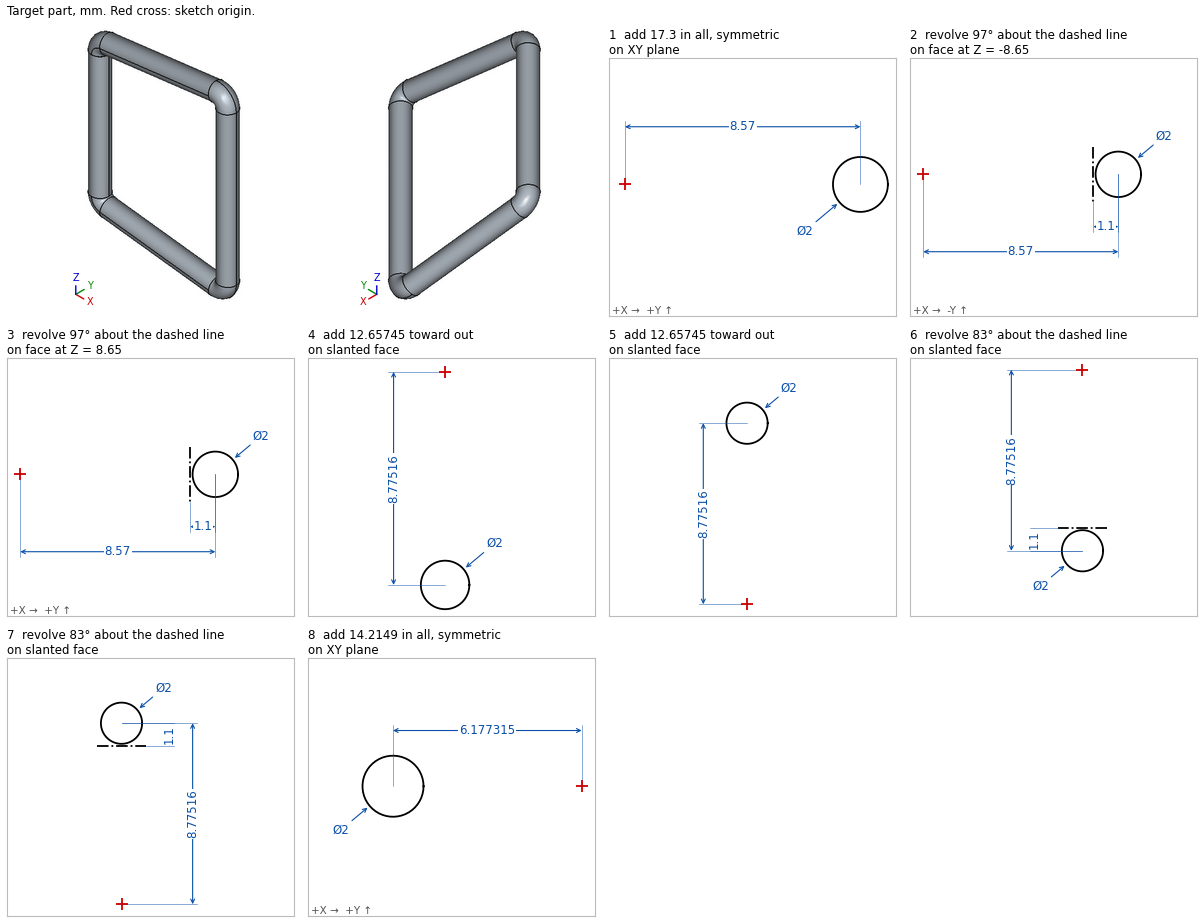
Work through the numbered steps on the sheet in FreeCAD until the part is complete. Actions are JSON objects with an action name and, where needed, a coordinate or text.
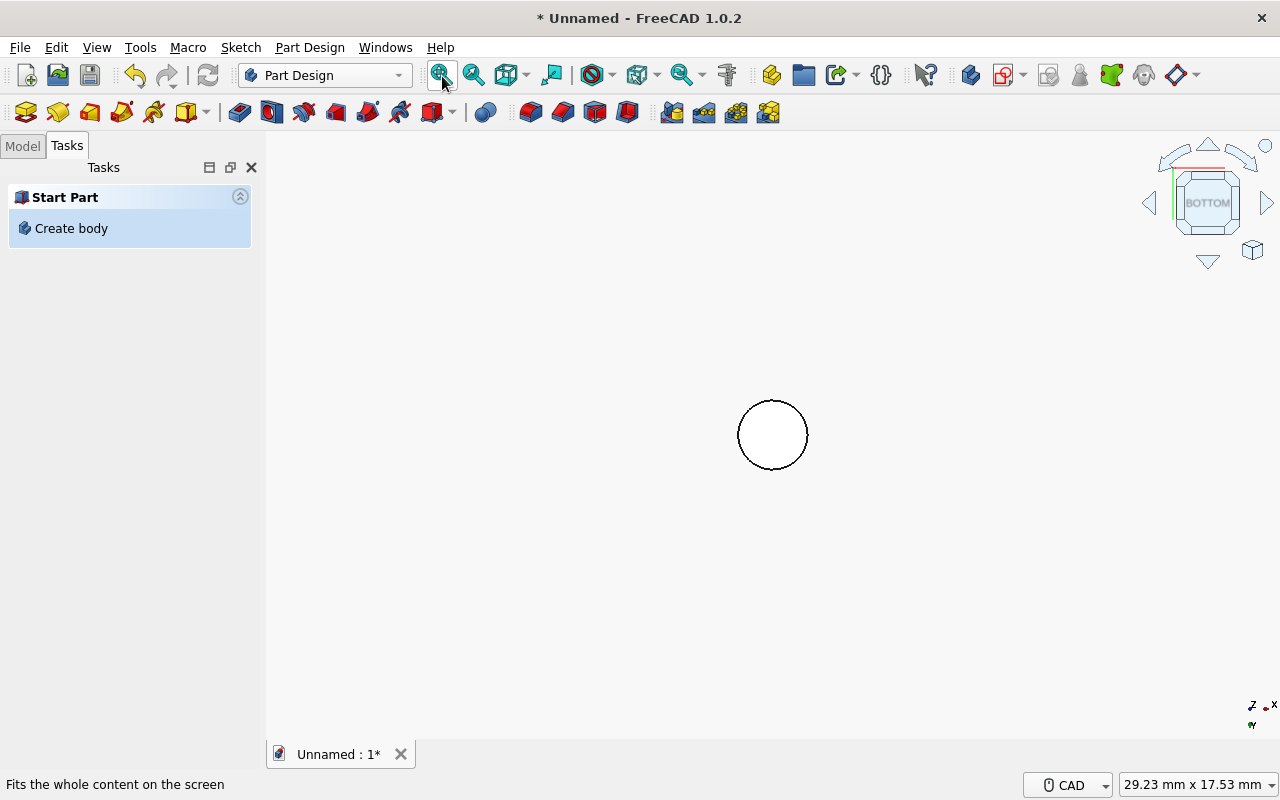
{"action": "left_click", "coordinate": [773, 434]}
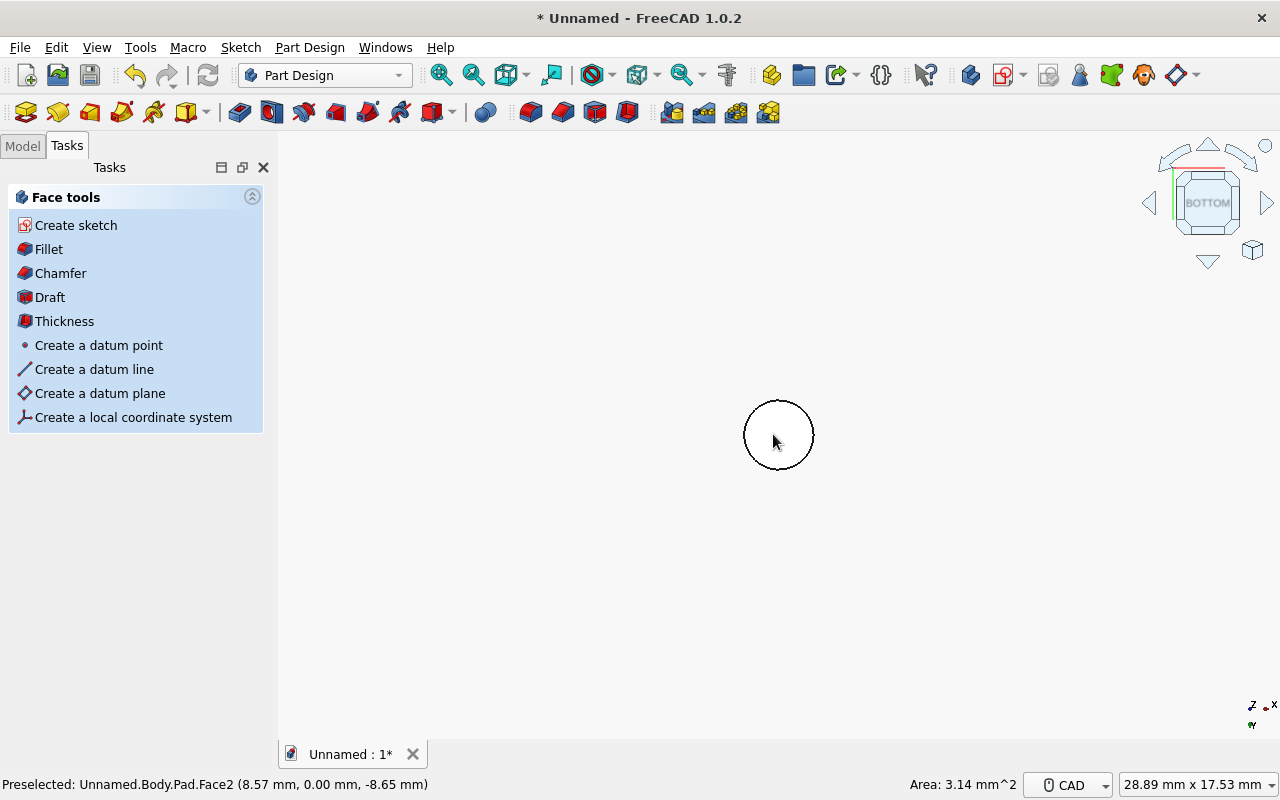
{"action": "left_click", "coordinate": [1004, 76]}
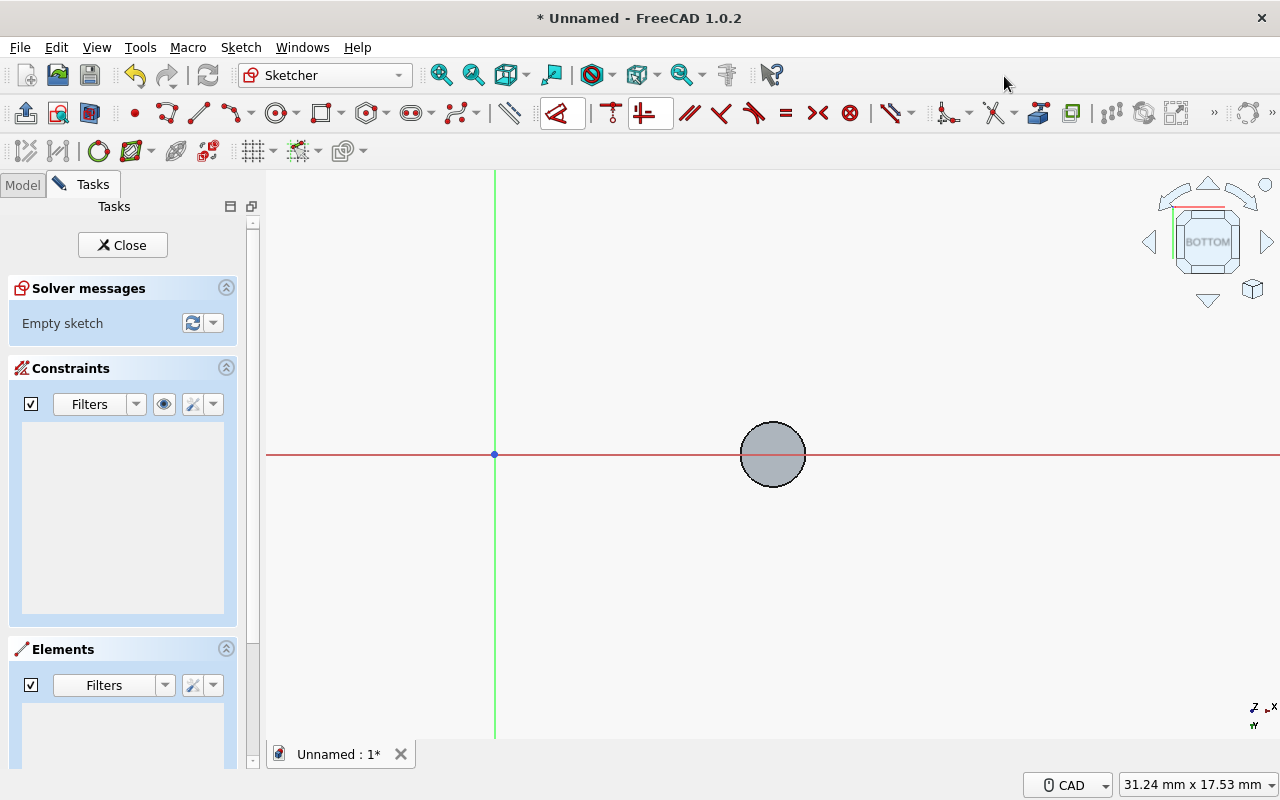
{"action": "scroll", "coordinate": [788, 454], "scroll_direction": "up", "scroll_amount": 8}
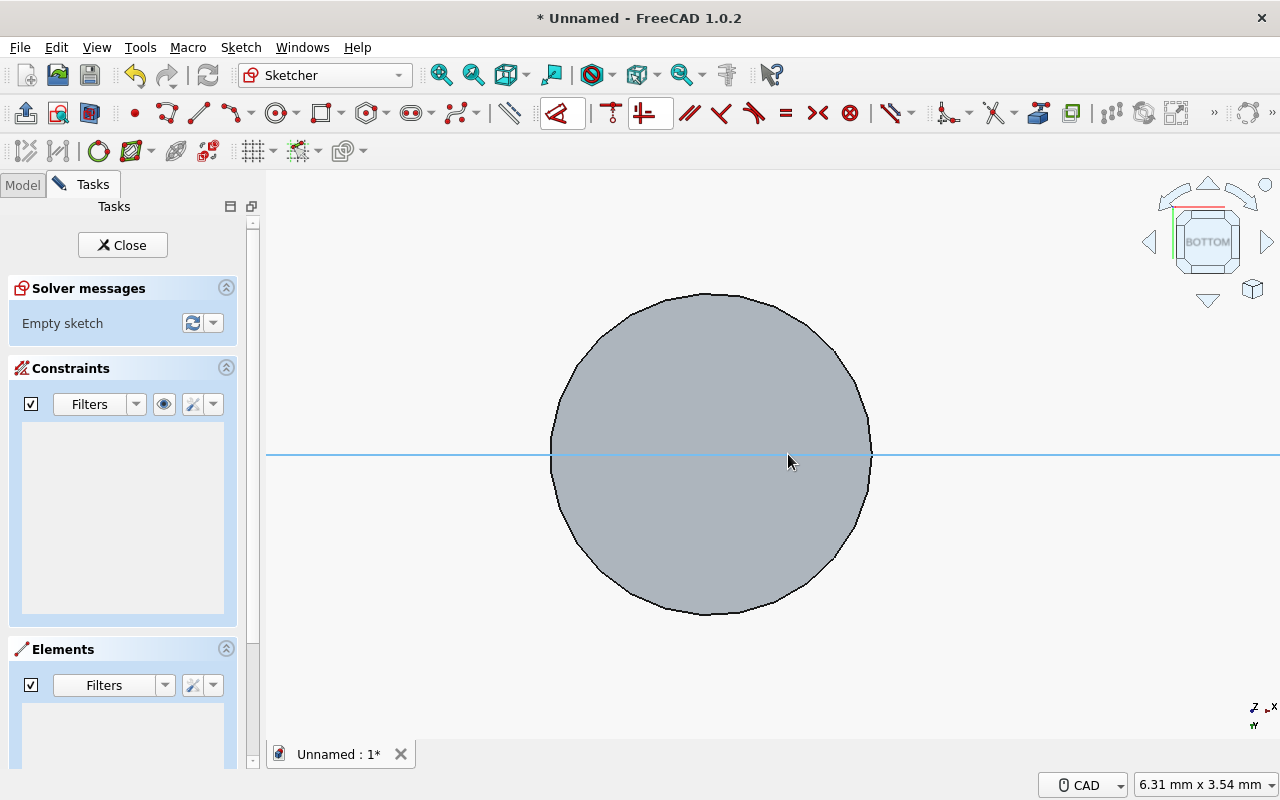
{"action": "key", "text": "g c"}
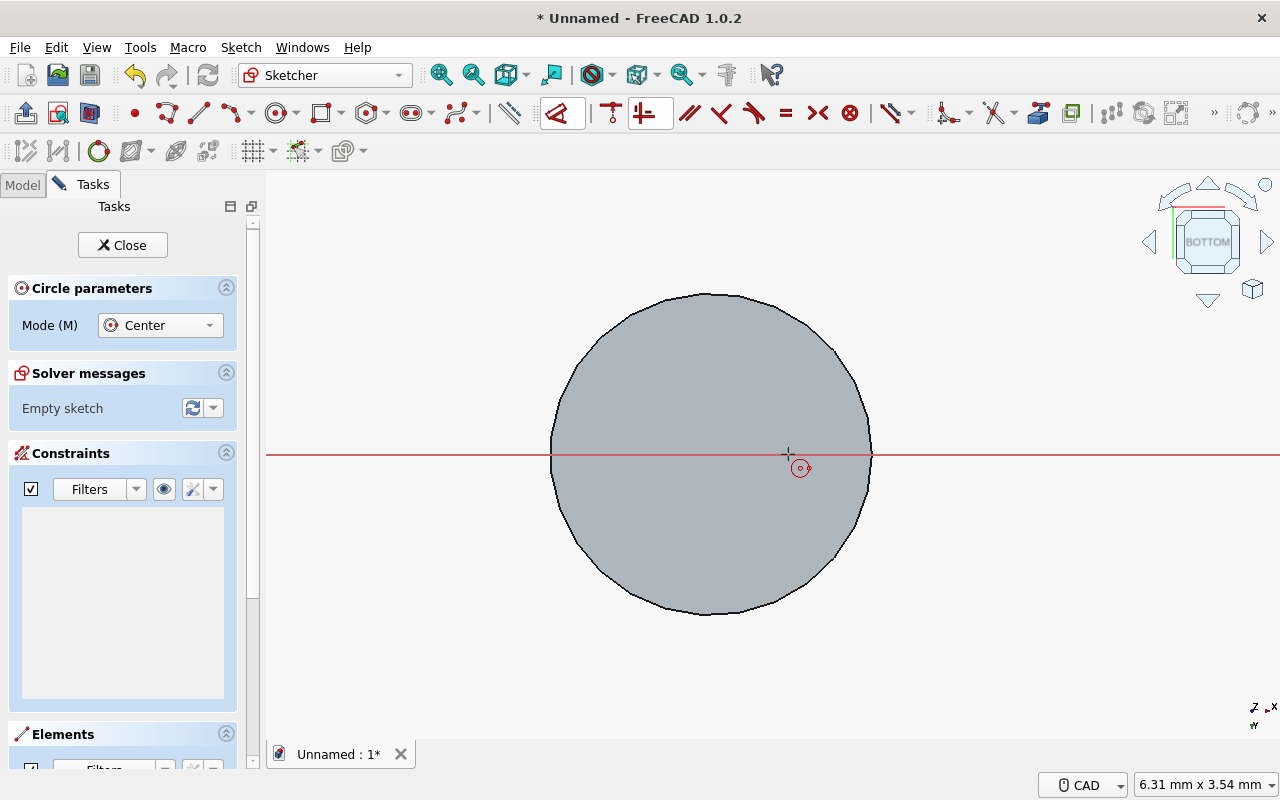
{"action": "left_click", "coordinate": [711, 454]}
{"action": "mouse_move", "coordinate": [825, 341]}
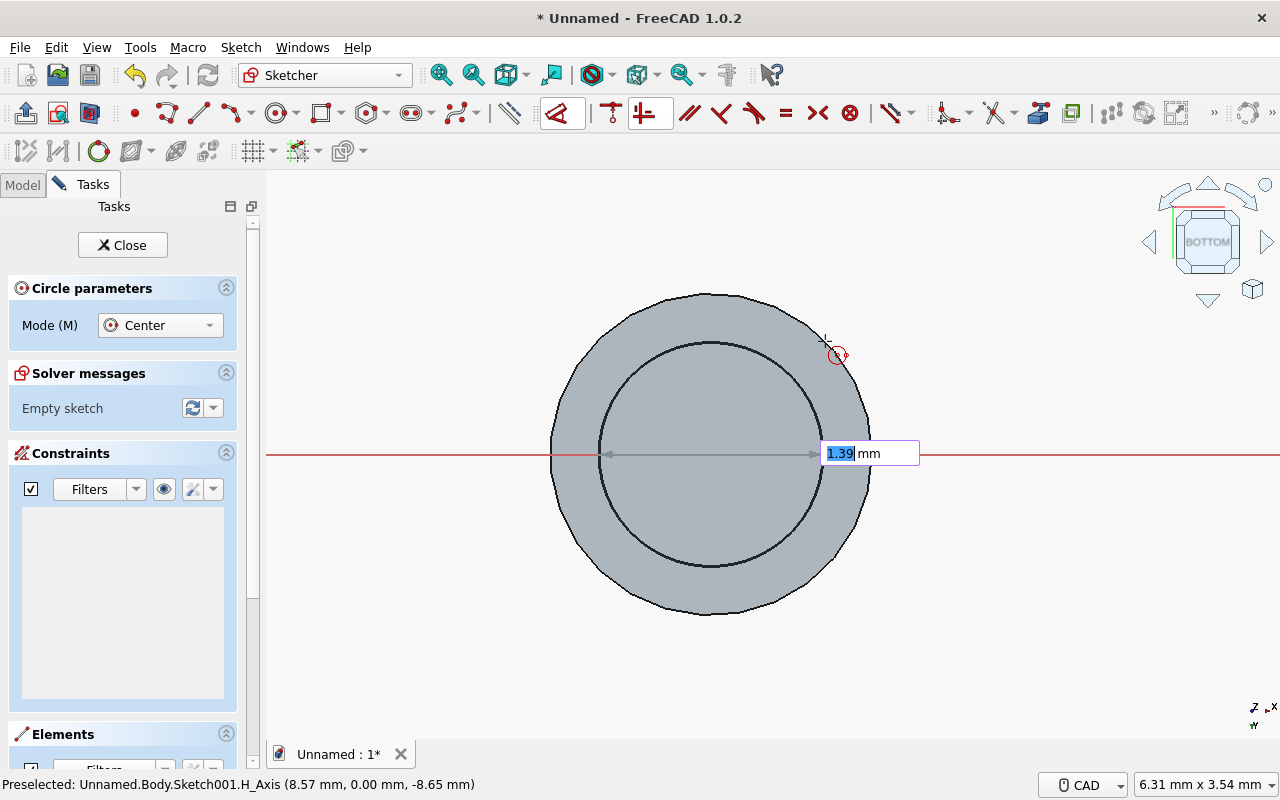
{"action": "type", "text": "2"}
{"action": "key", "text": "Return"}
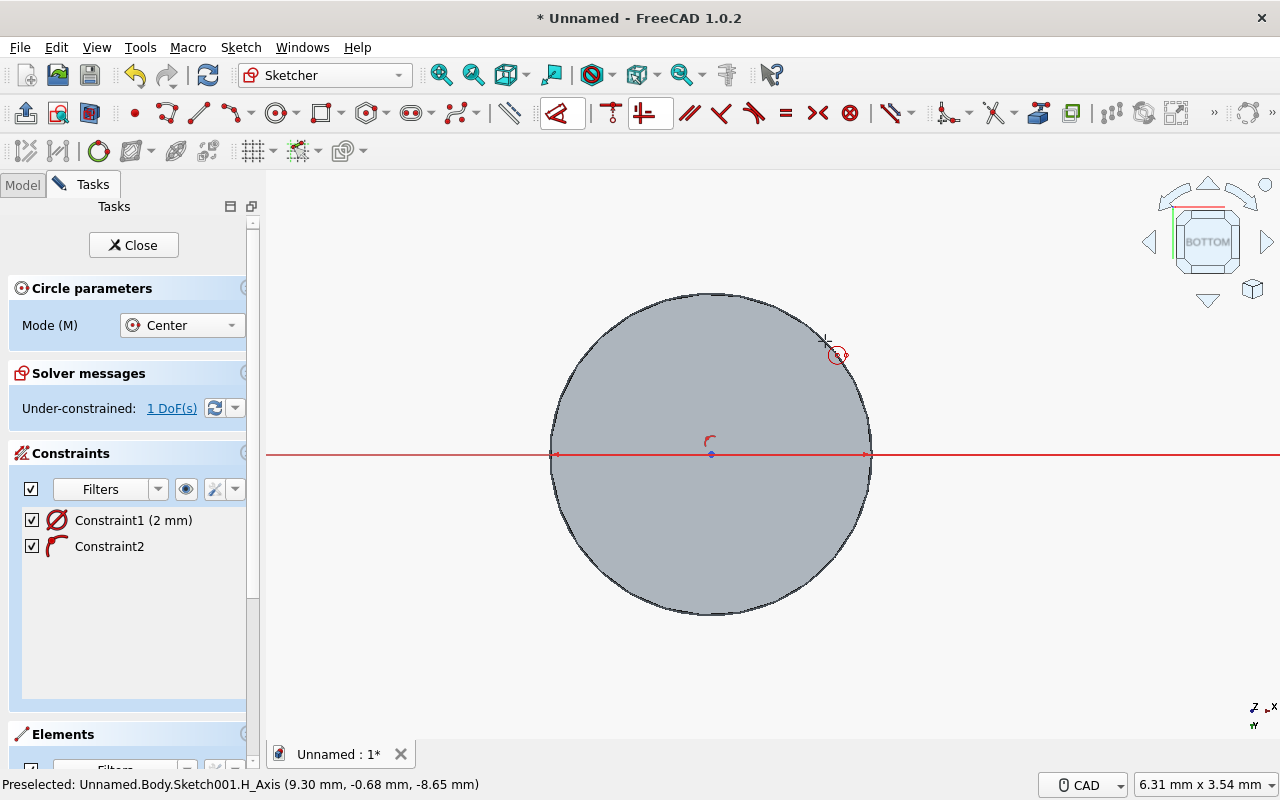
{"action": "left_click", "coordinate": [200, 114]}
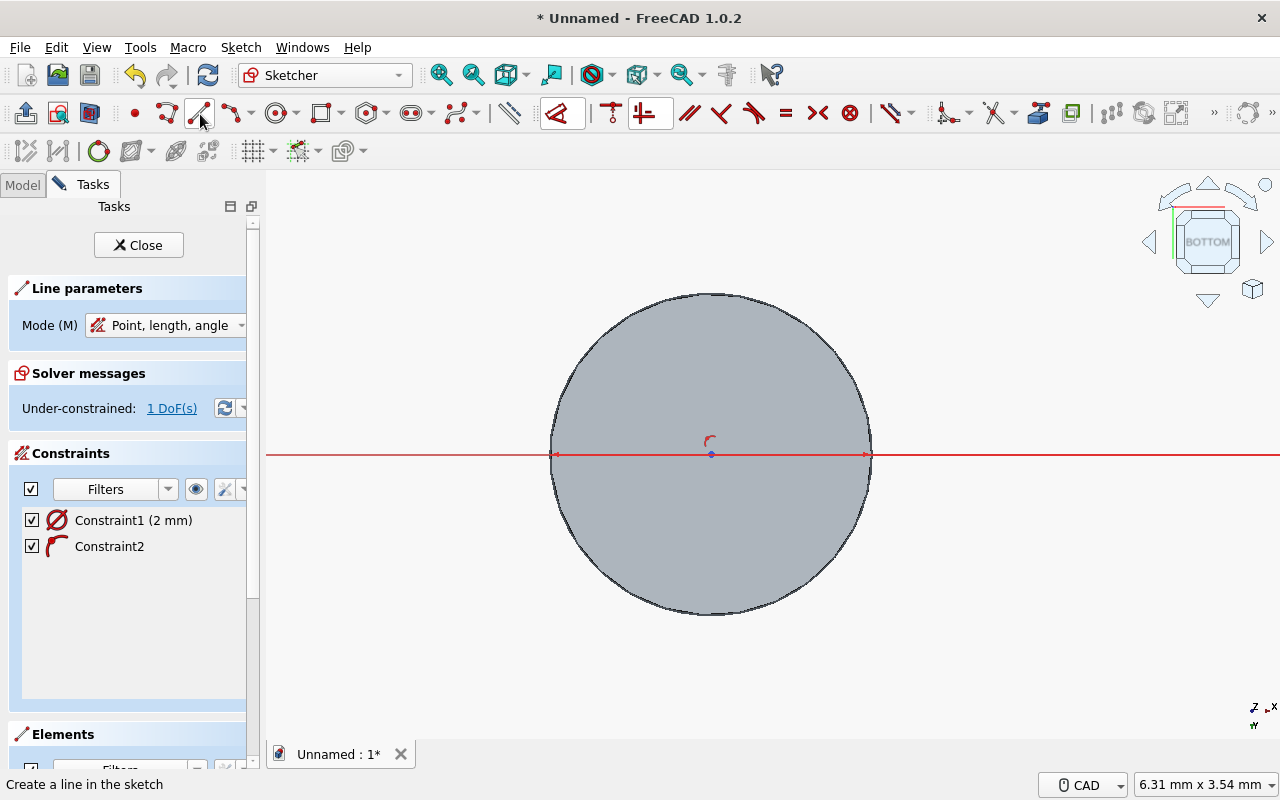
{"action": "left_click", "coordinate": [534, 262]}
{"action": "left_click", "coordinate": [534, 647]}
{"action": "key", "text": "Escape"}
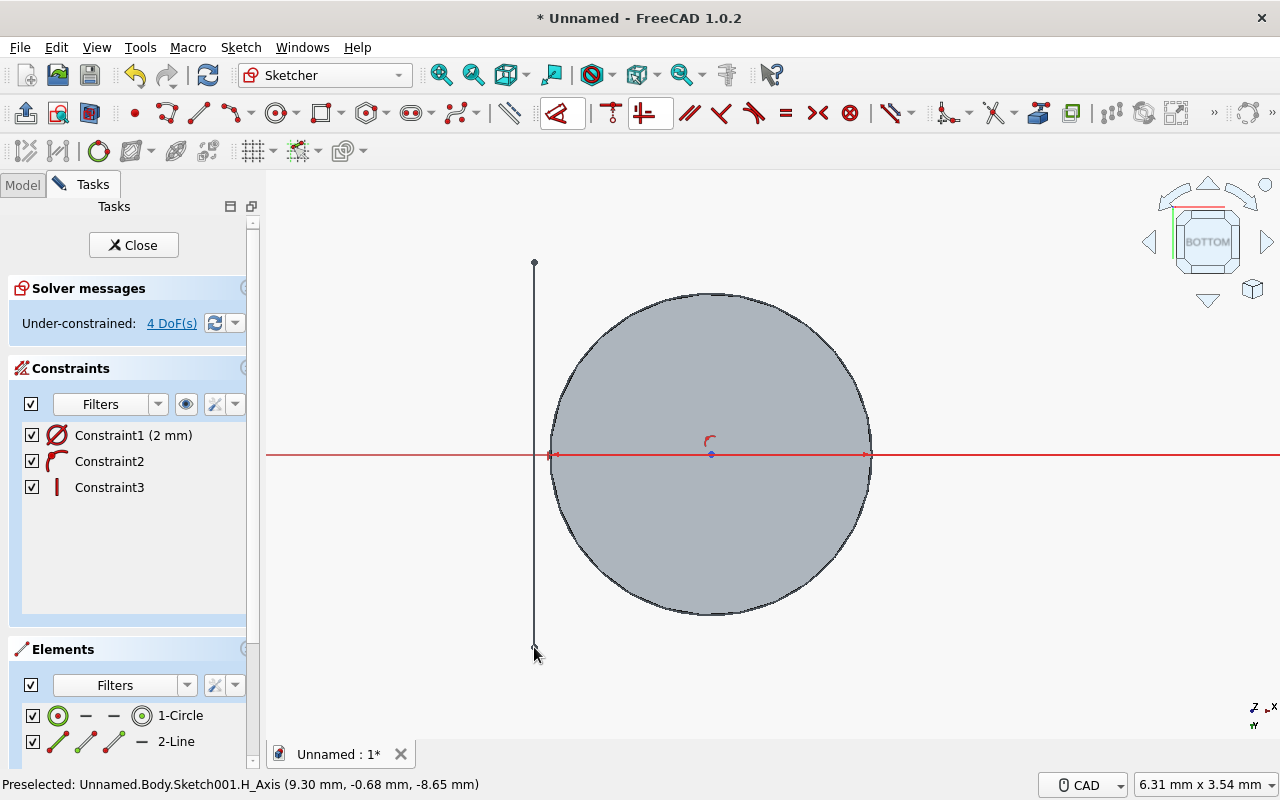
{"action": "left_click", "coordinate": [534, 378]}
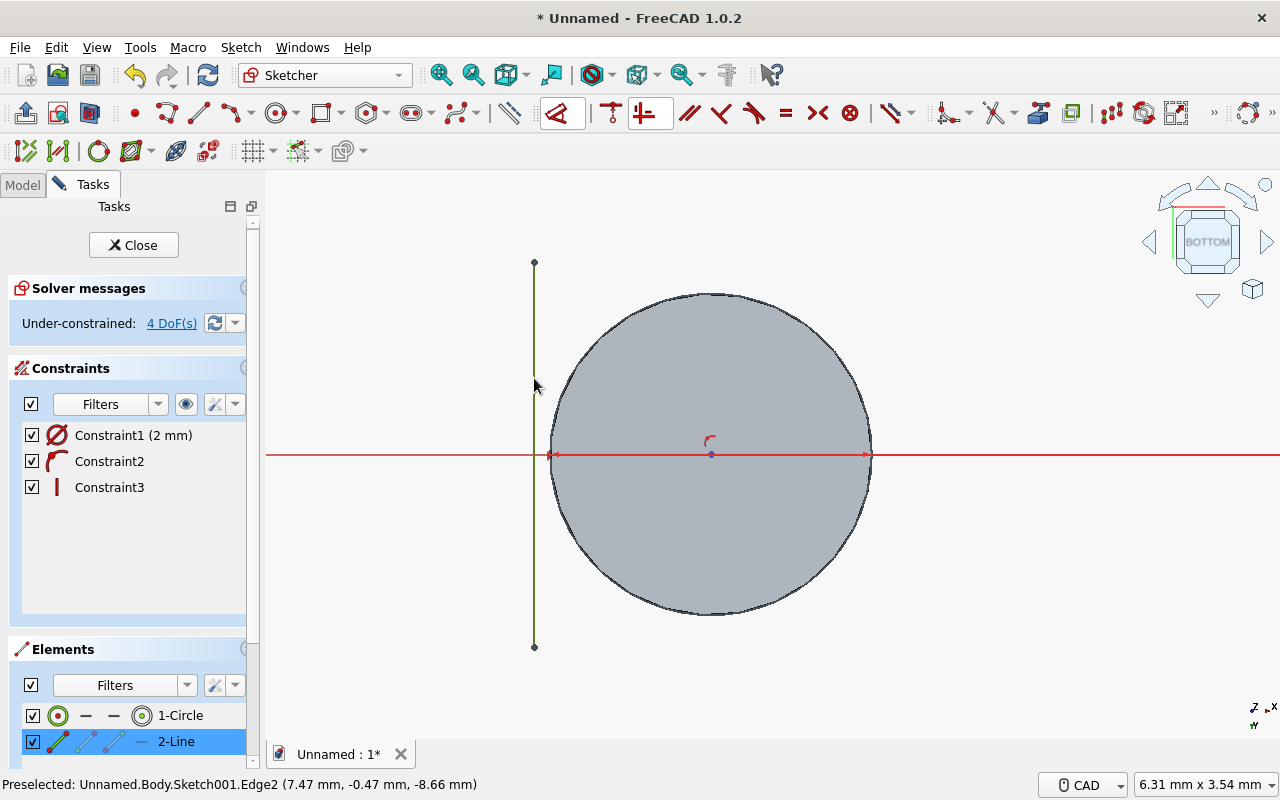
{"action": "left_click", "coordinate": [510, 114]}